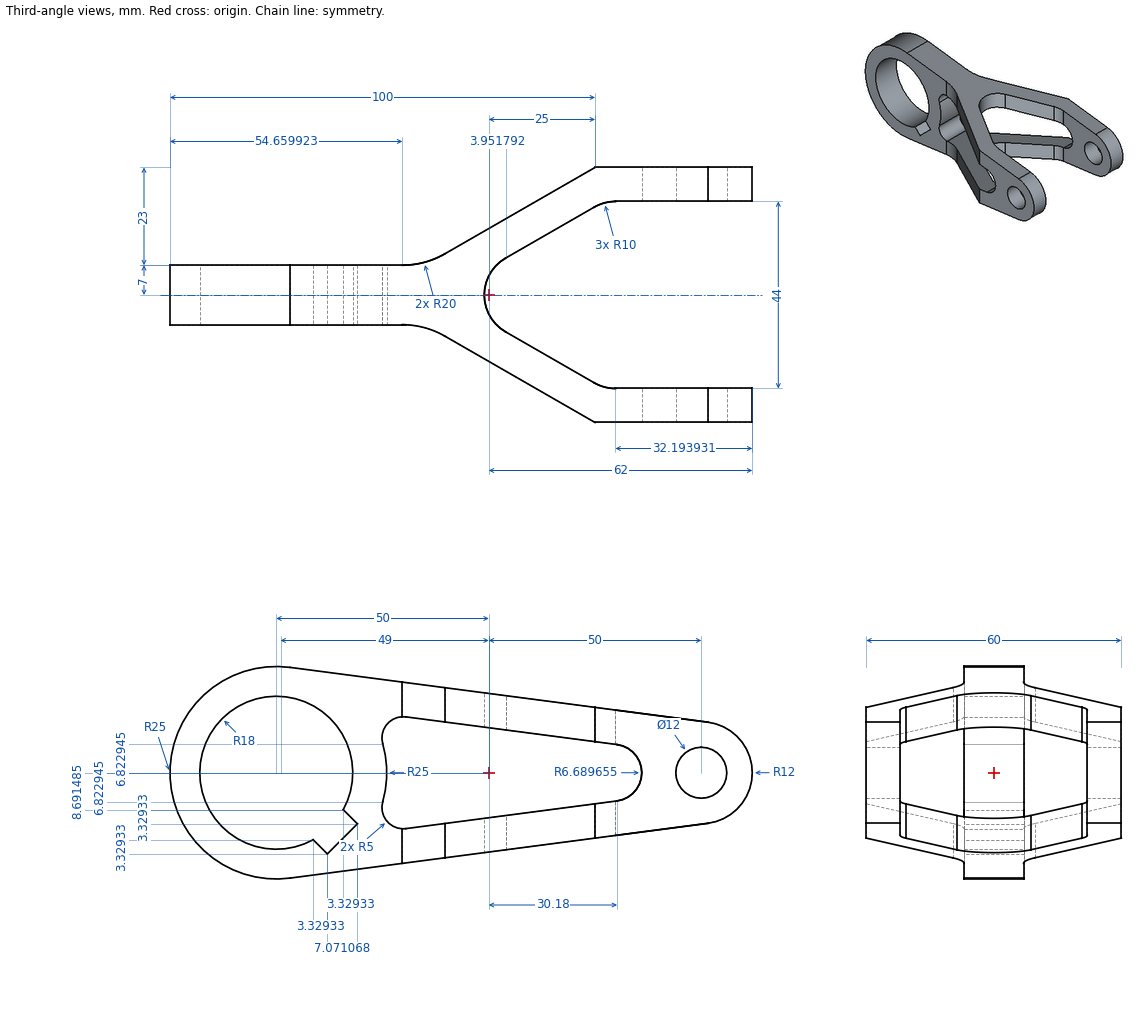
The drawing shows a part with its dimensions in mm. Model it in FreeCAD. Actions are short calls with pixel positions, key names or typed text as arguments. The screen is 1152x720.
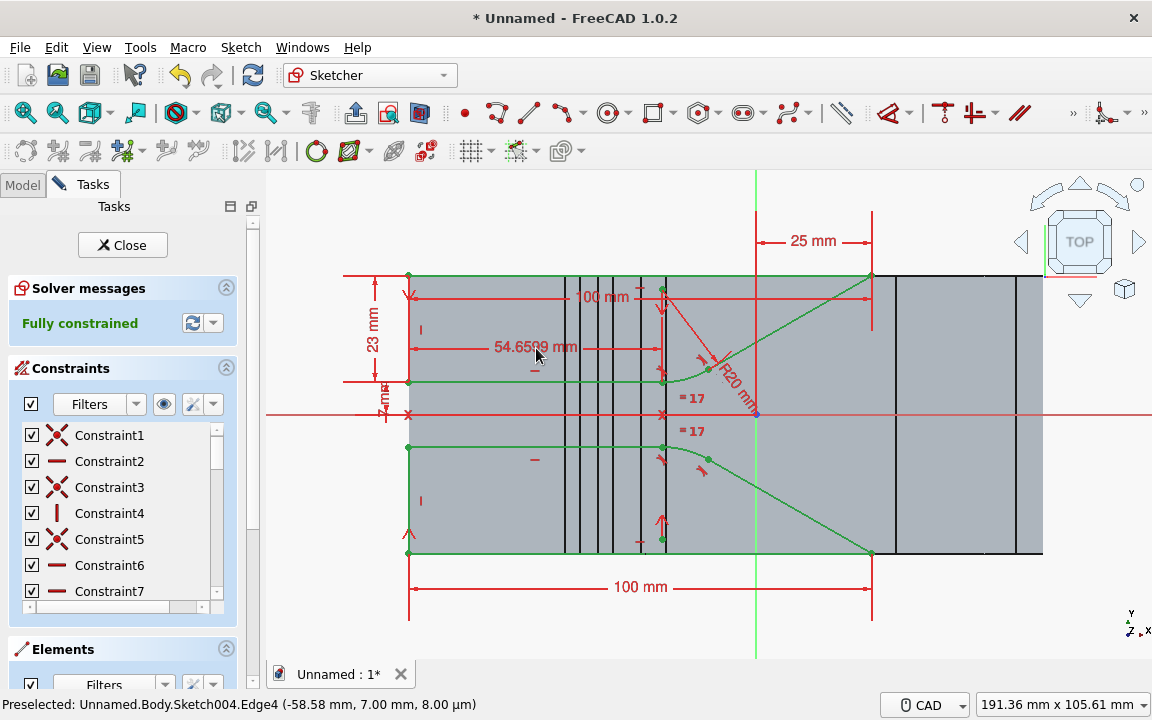
click(123, 245)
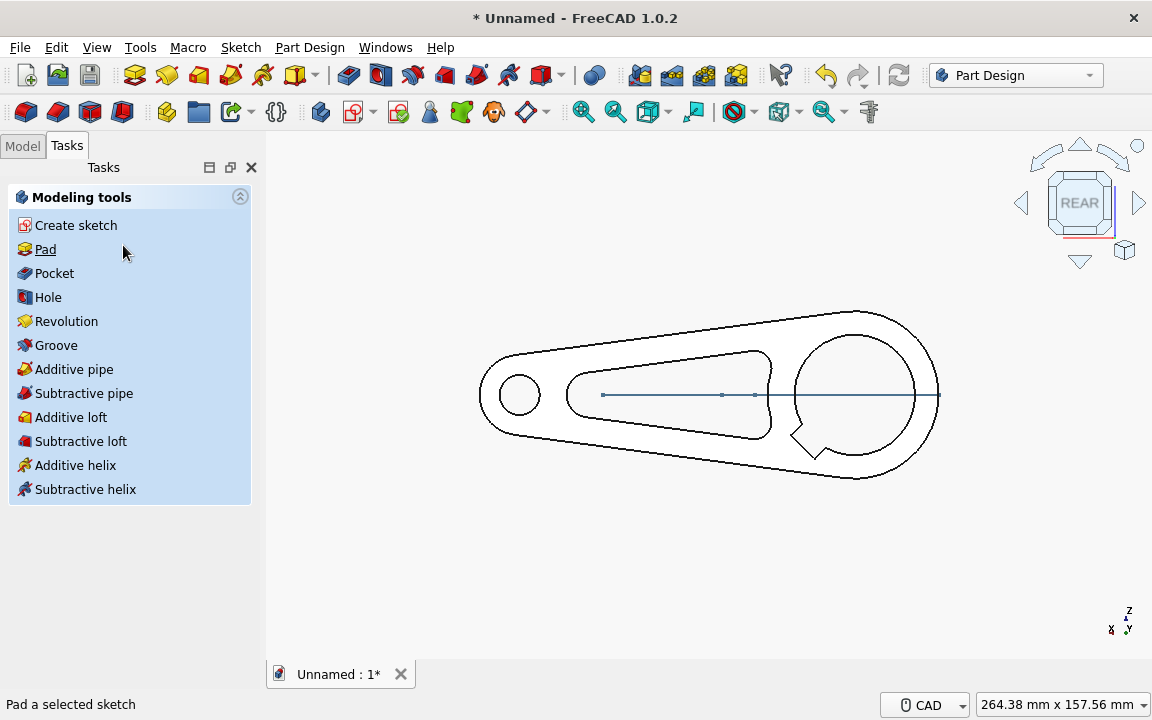
click(350, 76)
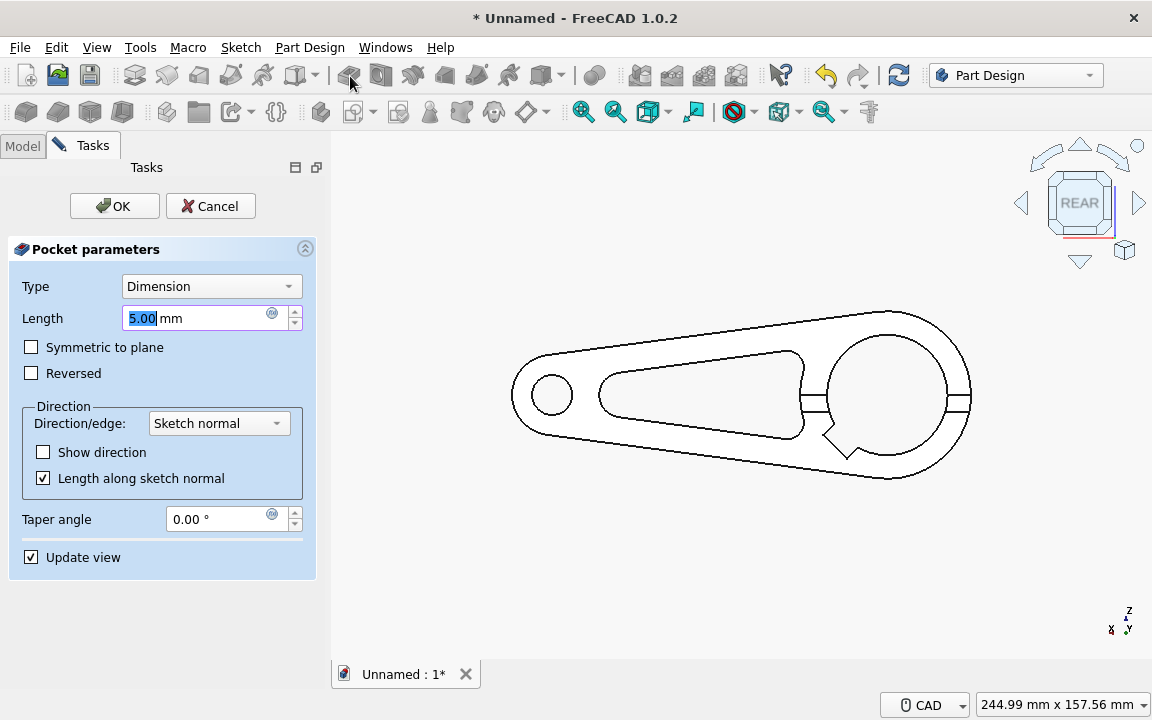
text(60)
key(Tab)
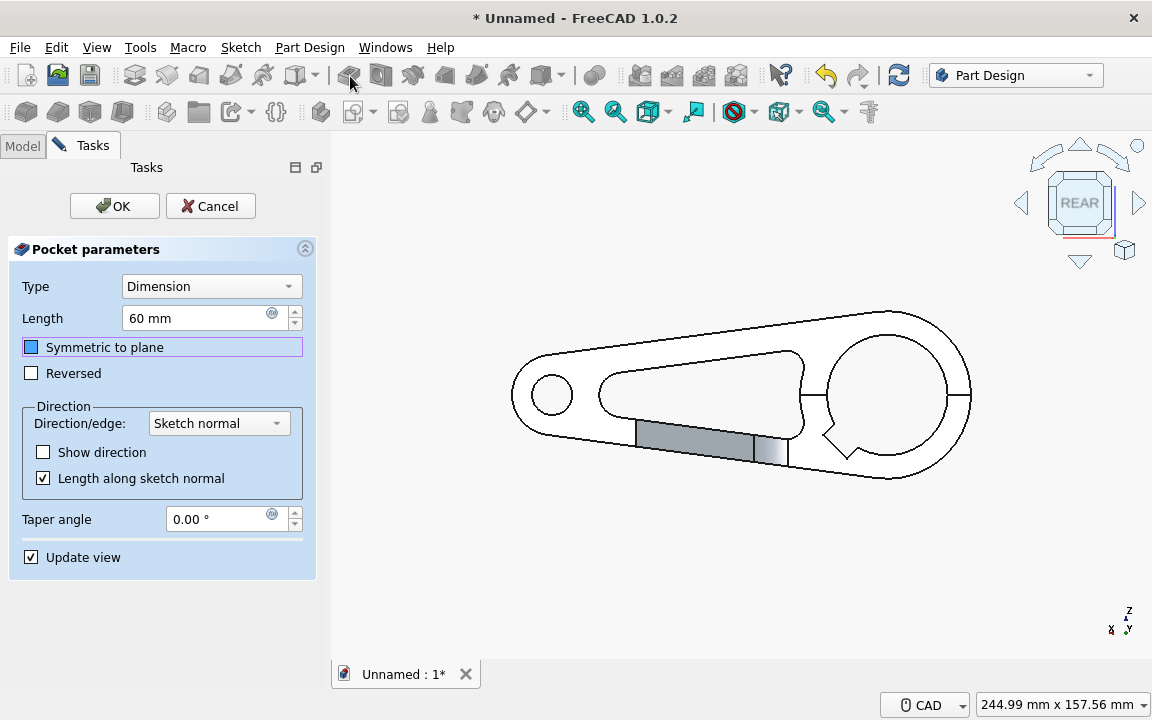
click(30, 347)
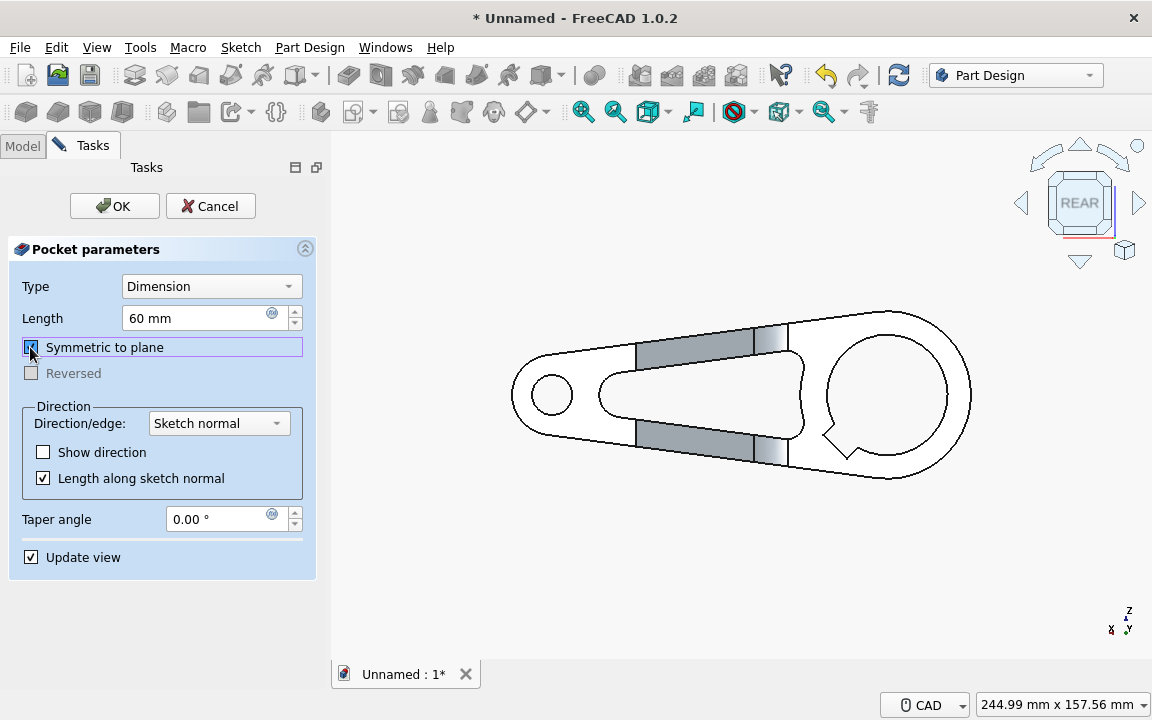
click(115, 206)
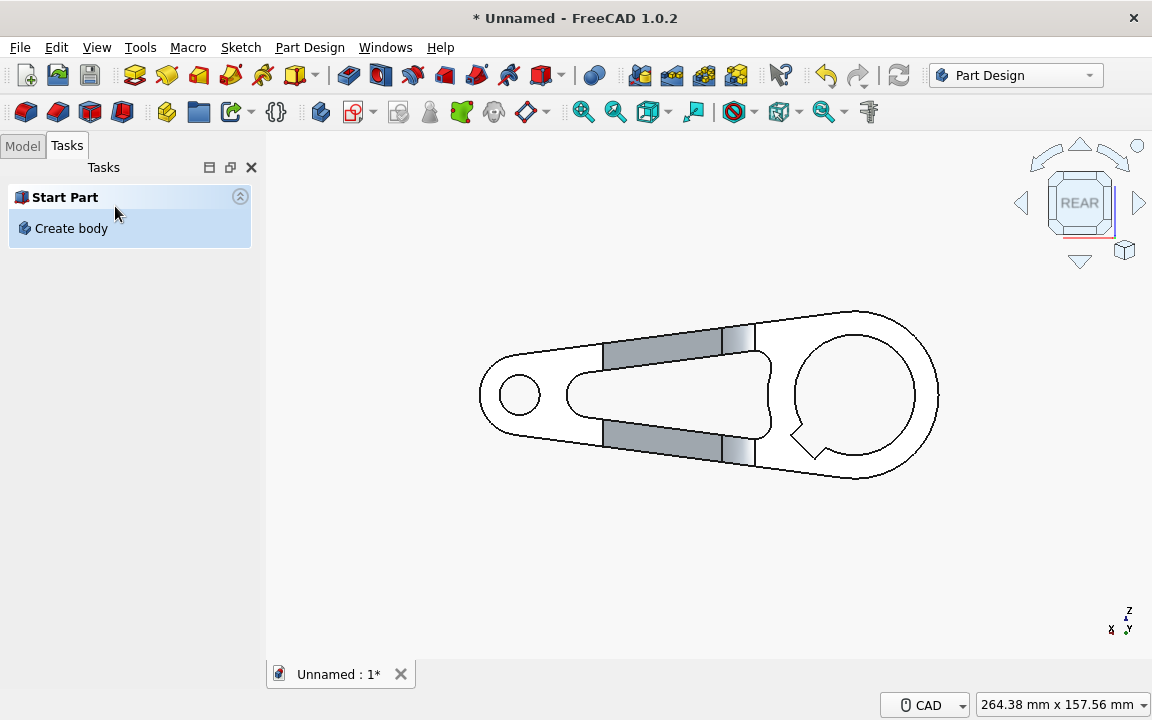
click(354, 112)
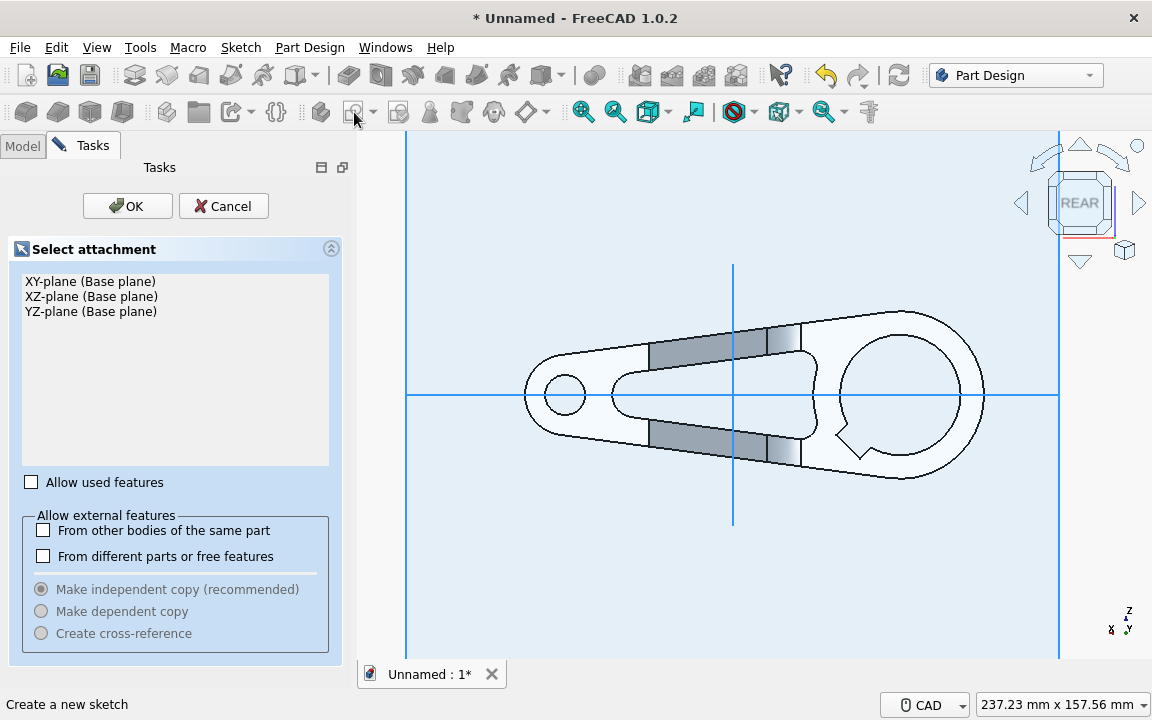
click(82, 282)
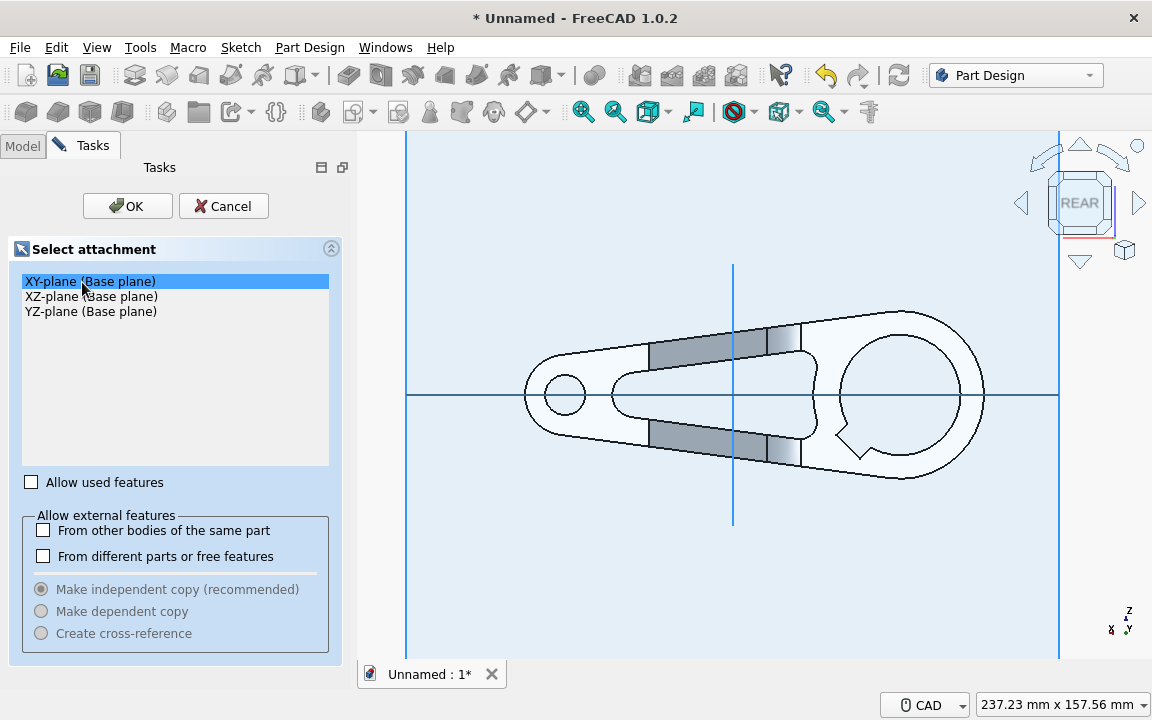
click(128, 206)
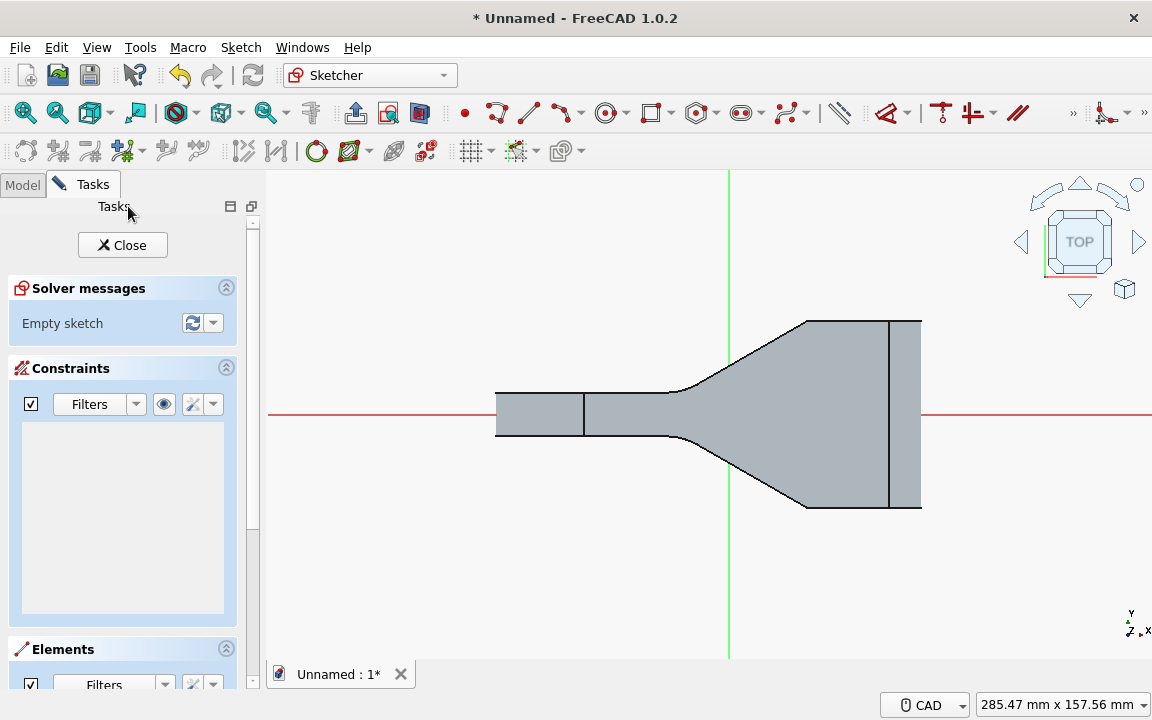
click(420, 114)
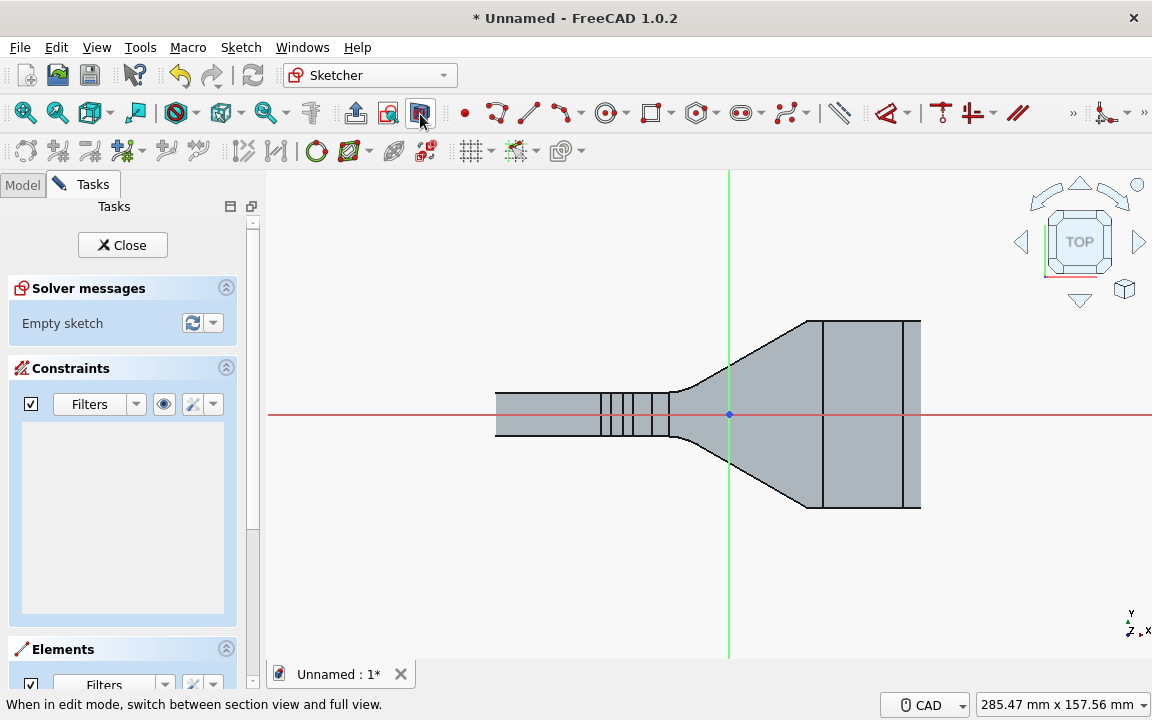
scroll(973, 414, up, 4)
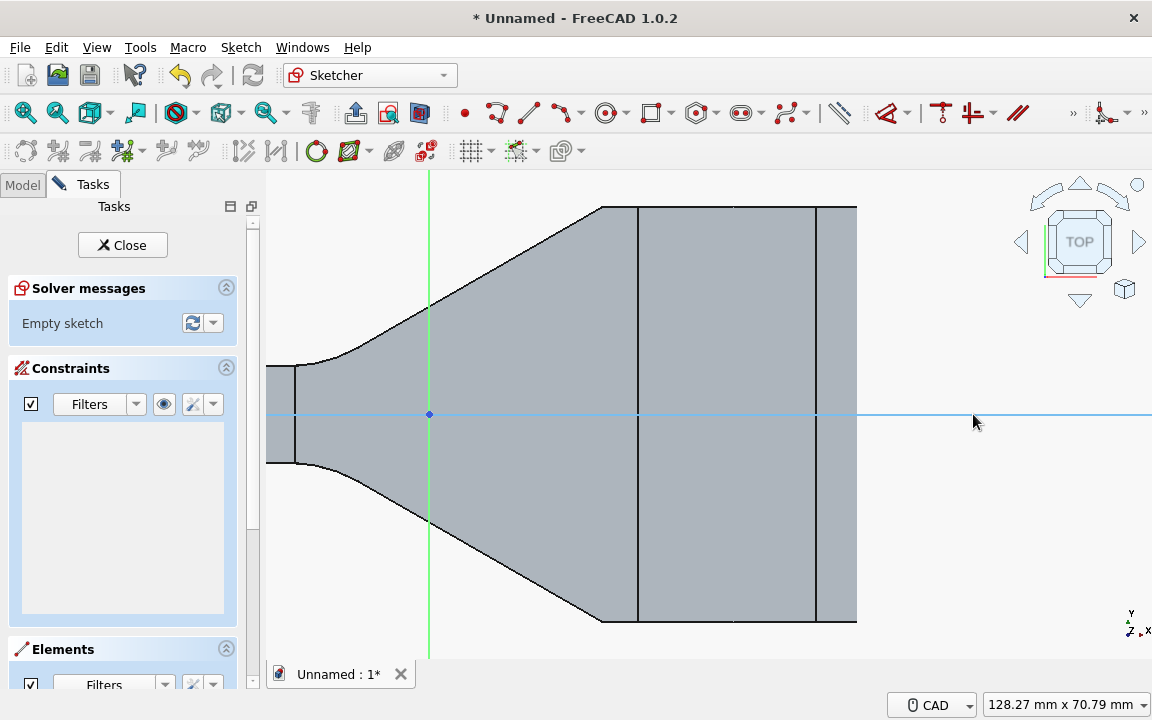
click(530, 114)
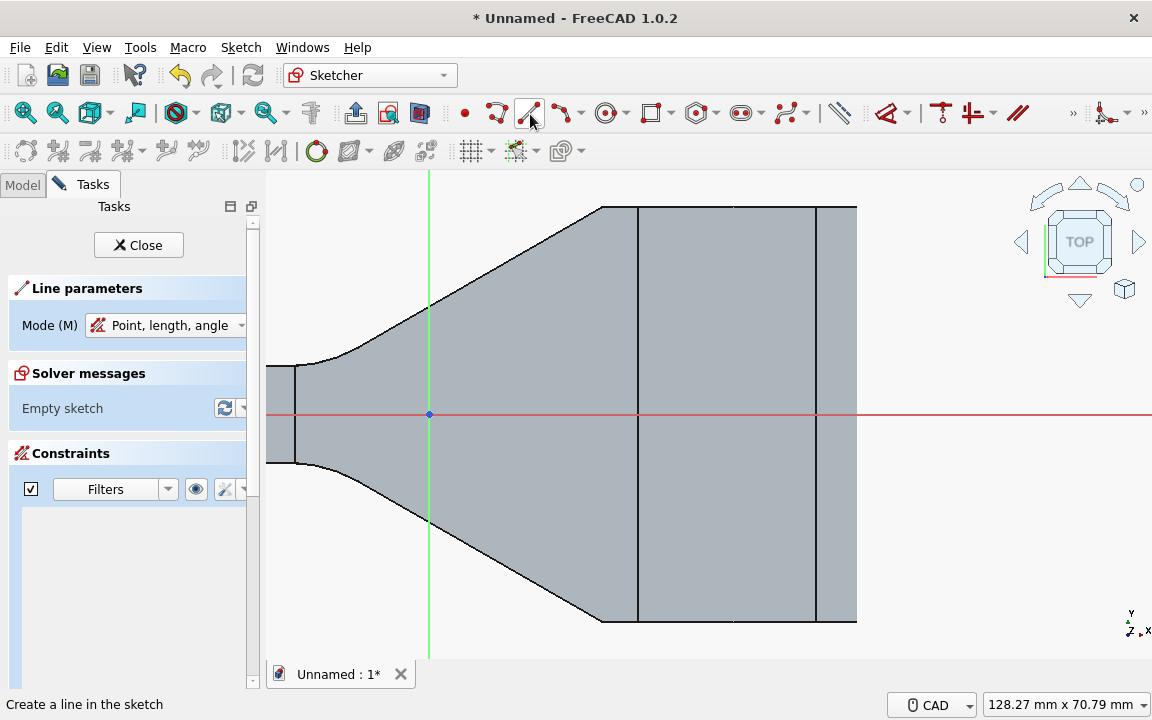
click(601, 272)
click(457, 355)